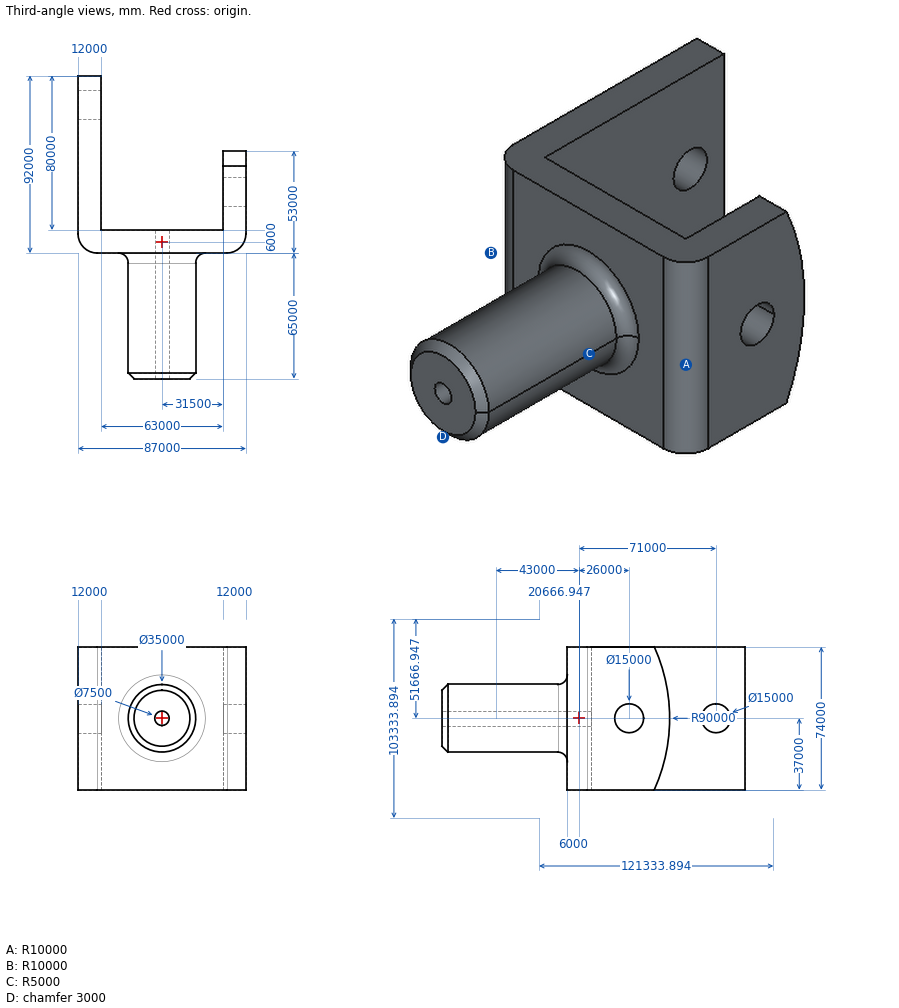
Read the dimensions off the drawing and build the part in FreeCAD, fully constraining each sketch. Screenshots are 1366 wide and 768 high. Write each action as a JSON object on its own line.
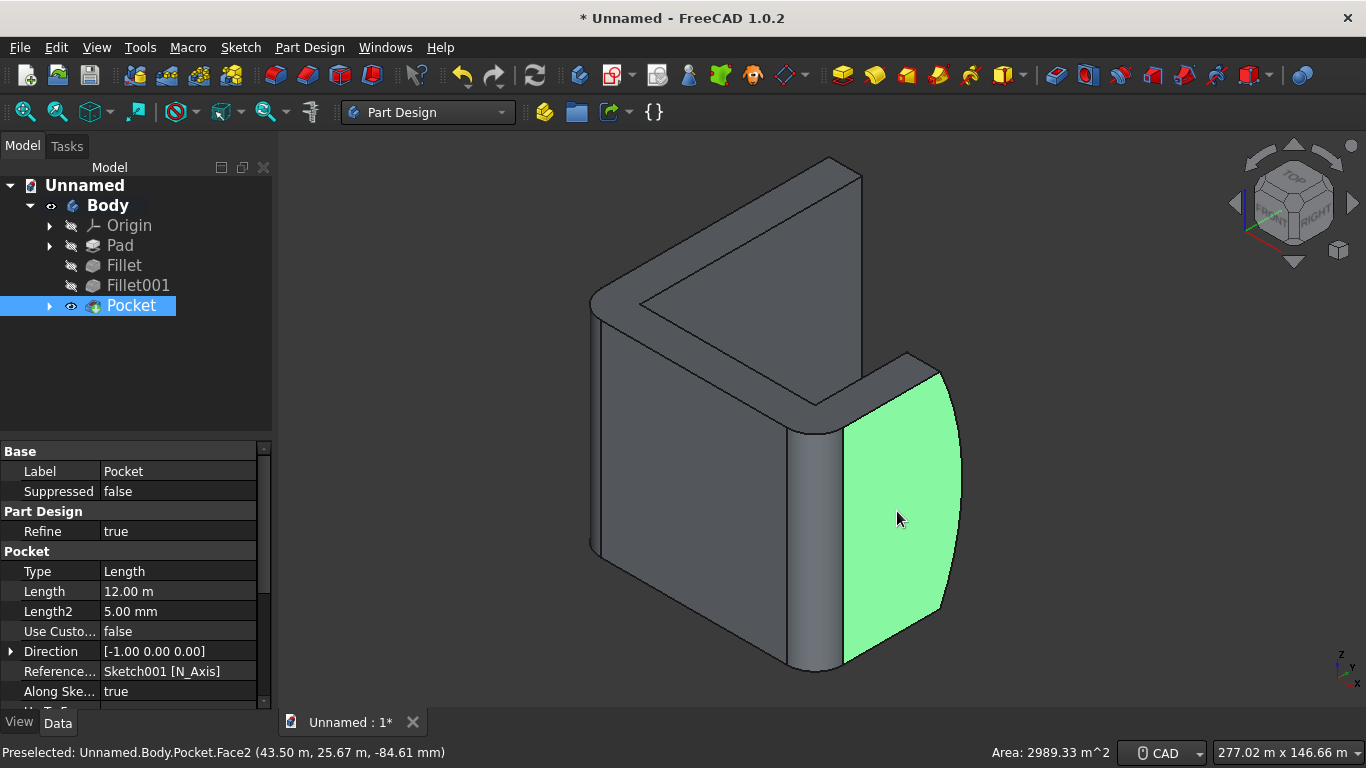
{"action": "left_click", "coordinate": [612, 76]}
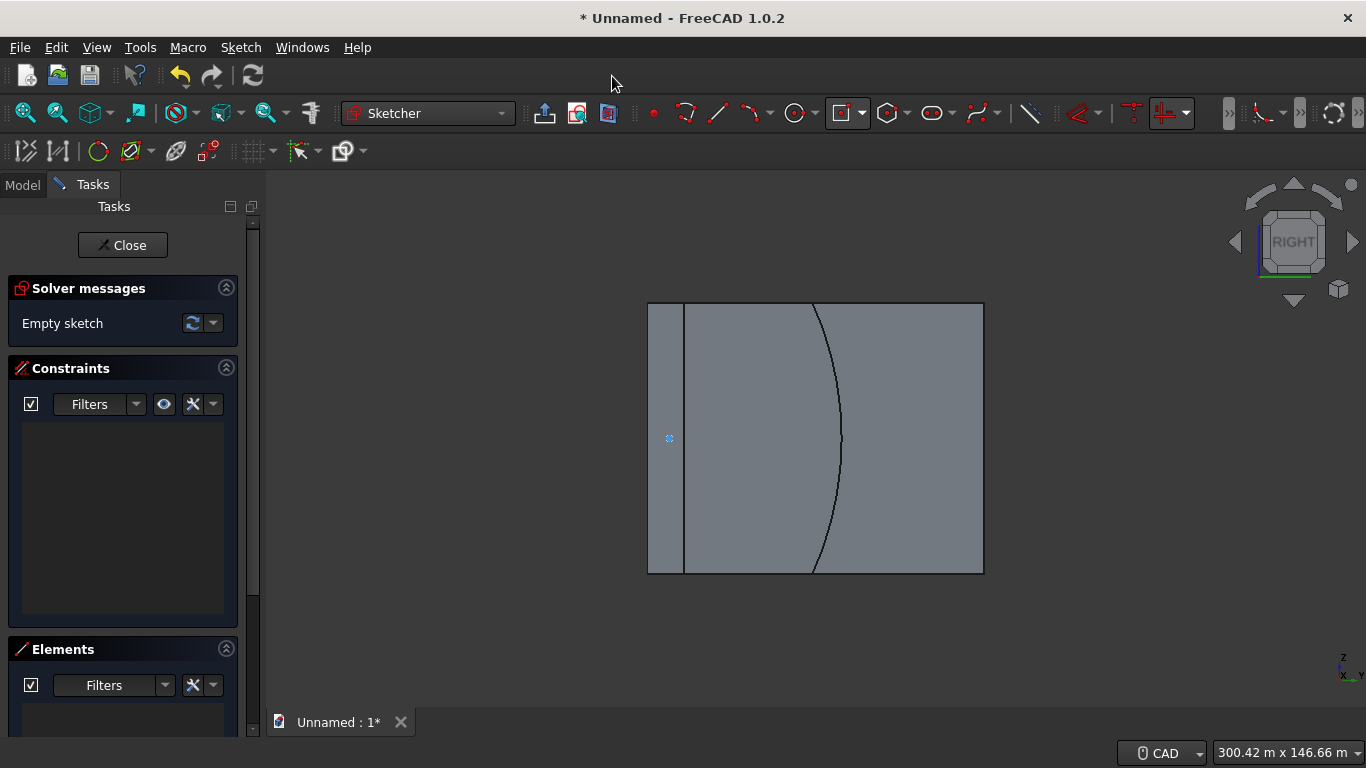
{"action": "scroll", "coordinate": [727, 438], "scroll_direction": "up", "scroll_amount": 8}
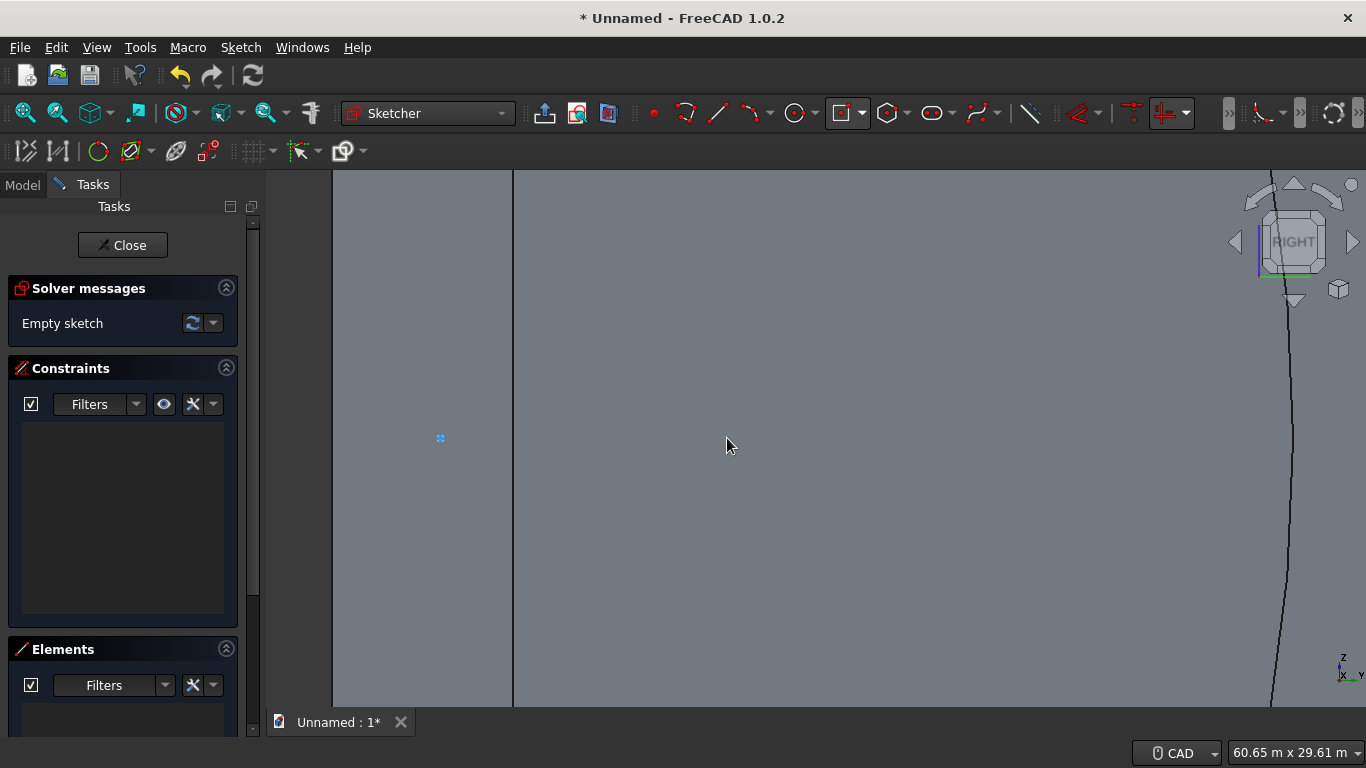
{"action": "left_click", "coordinate": [796, 114]}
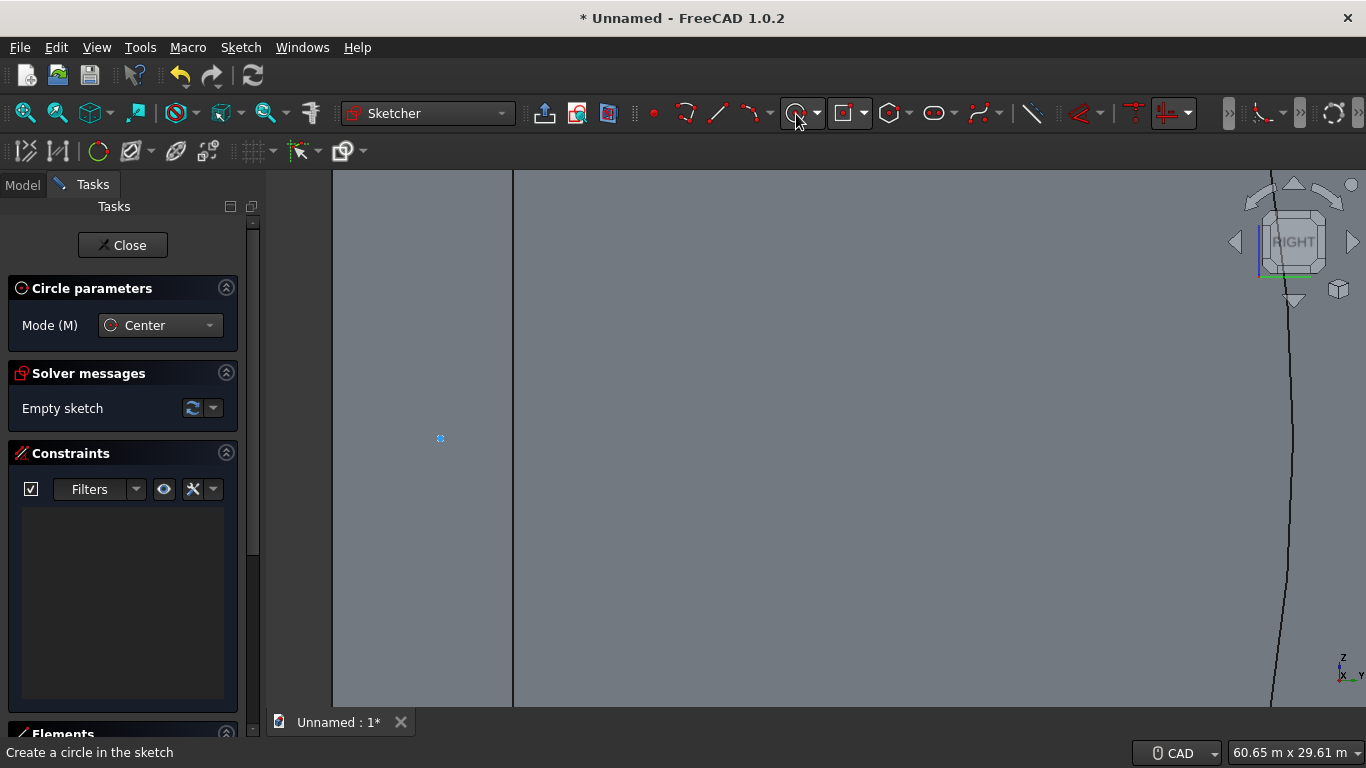
{"action": "left_click", "coordinate": [912, 438]}
{"action": "left_click", "coordinate": [1008, 342]}
{"action": "key", "text": "Escape"}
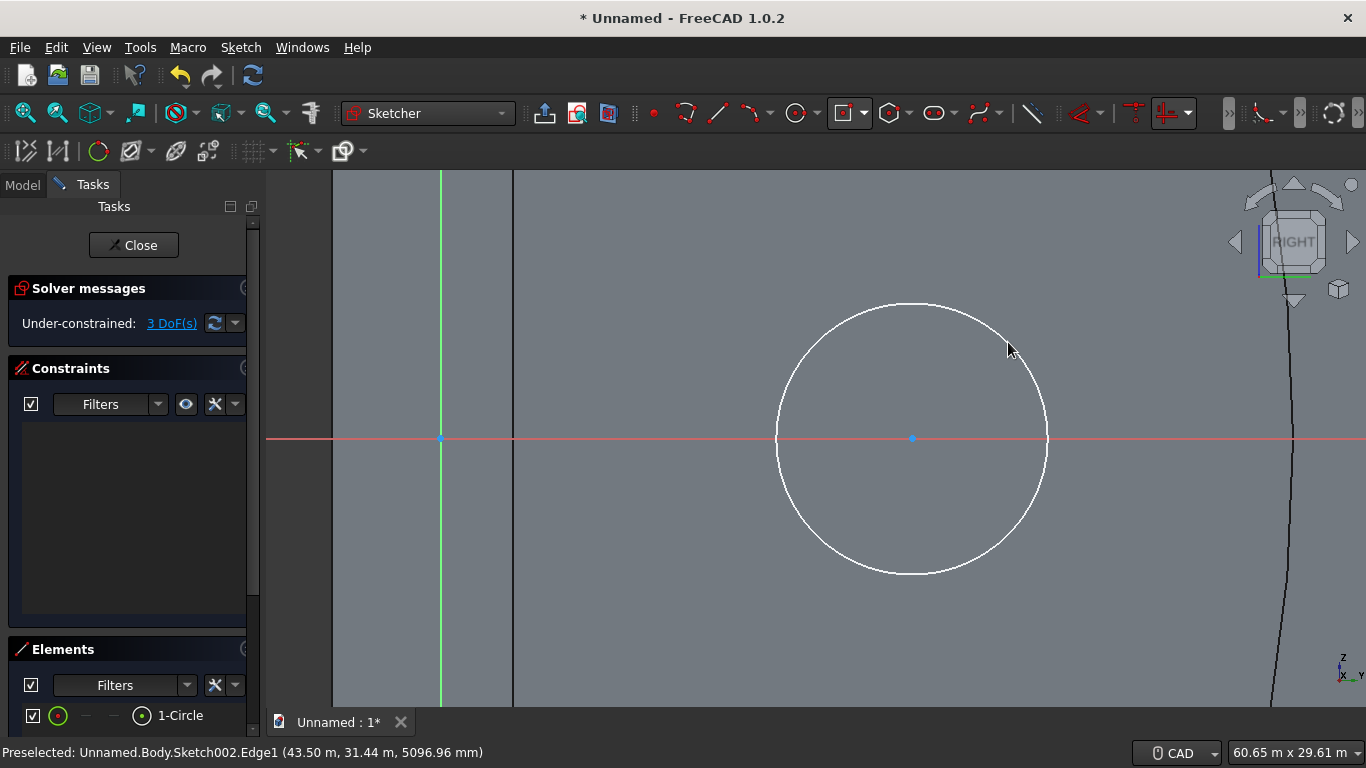
{"action": "left_click", "coordinate": [912, 439]}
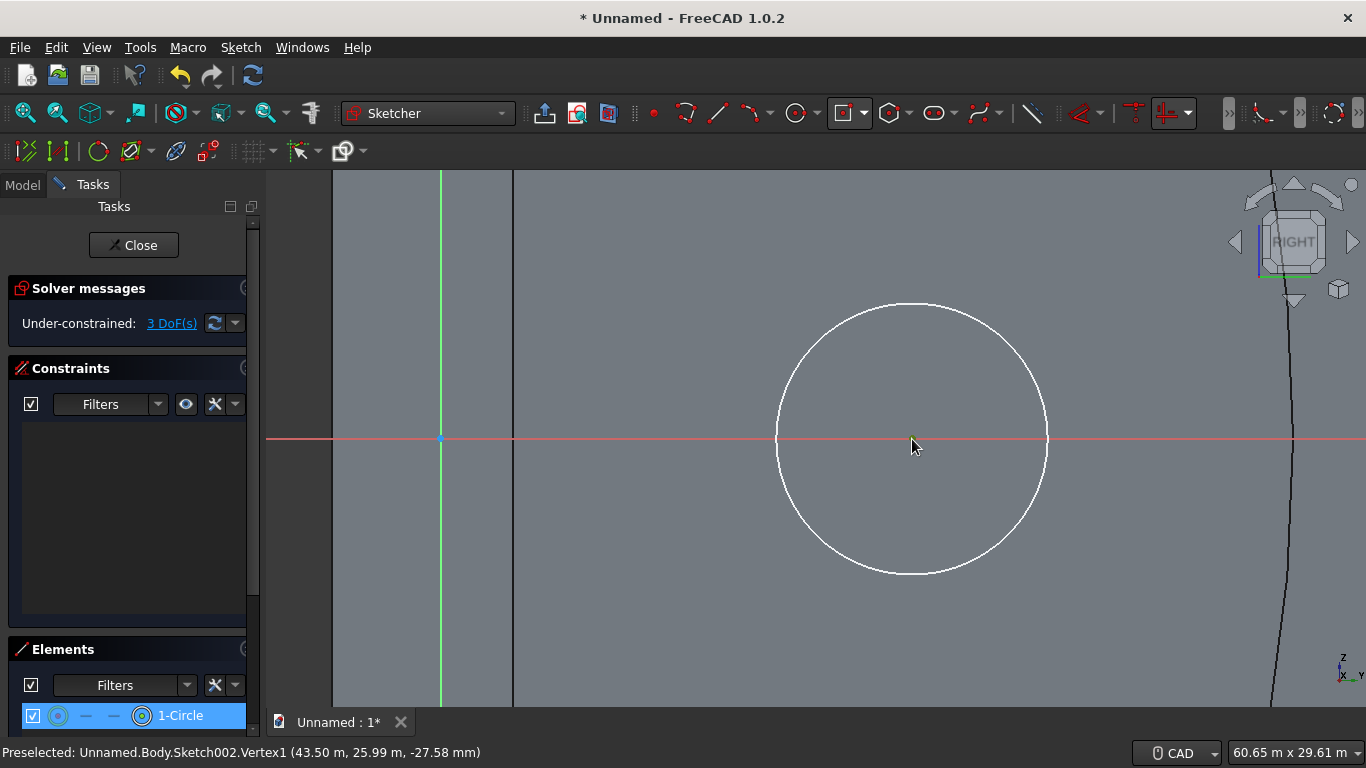
{"action": "left_click", "coordinate": [359, 438]}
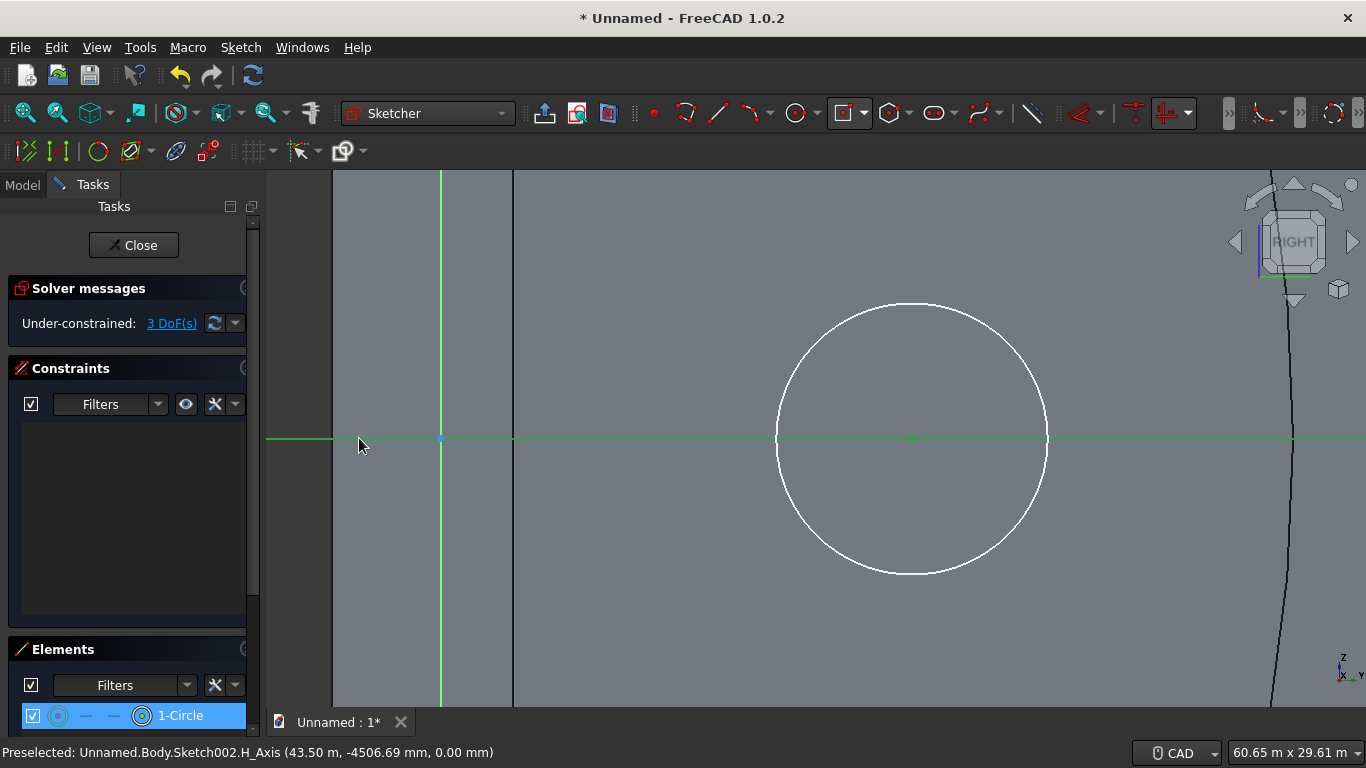
{"action": "left_click", "coordinate": [1134, 114]}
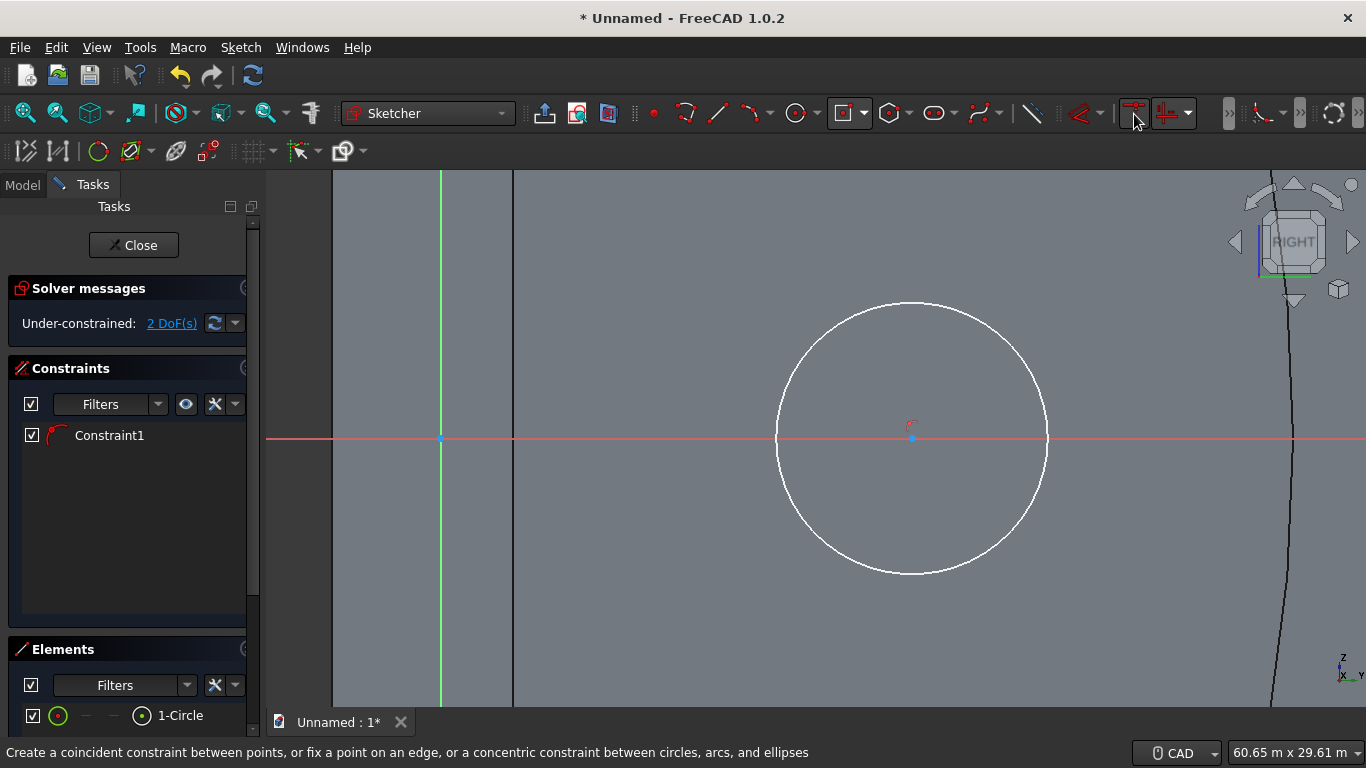
{"action": "left_click", "coordinate": [1080, 114]}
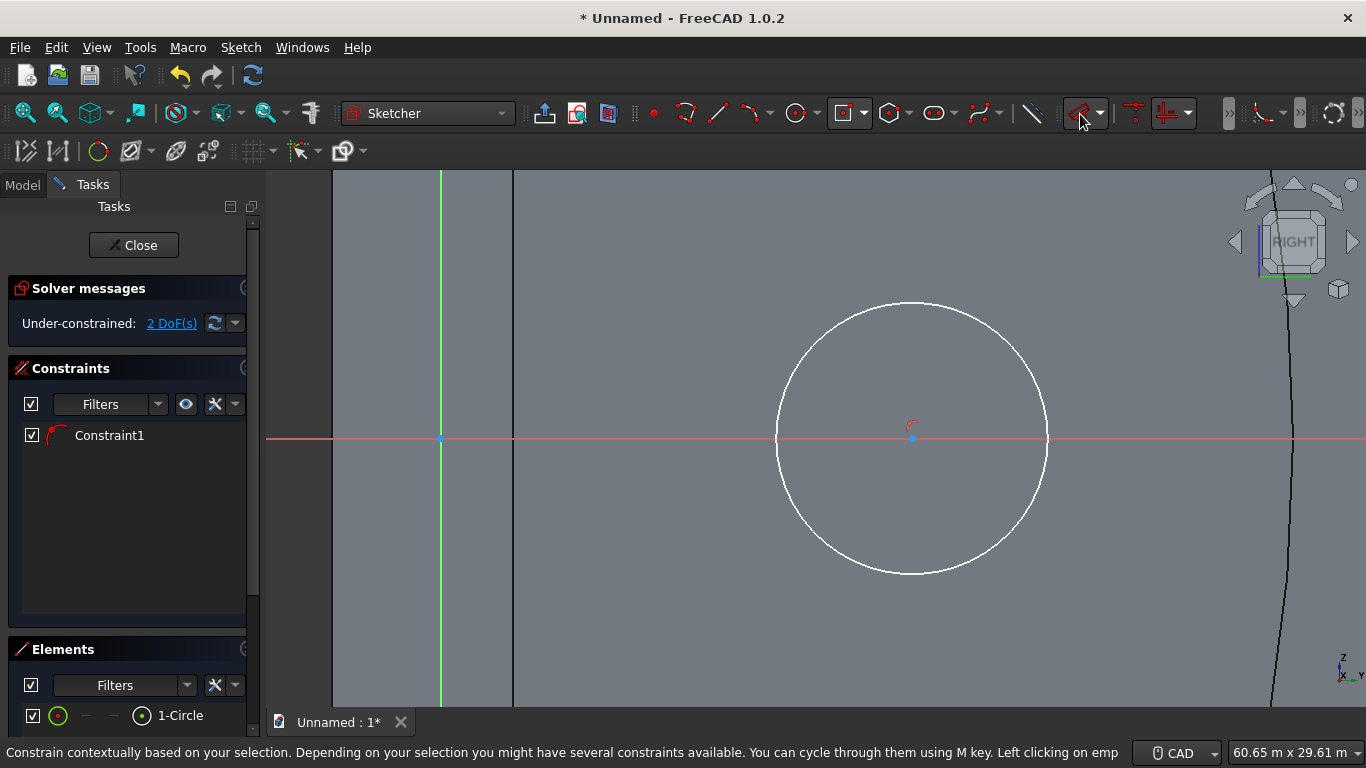
{"action": "left_click", "coordinate": [1008, 342]}
{"action": "left_click", "coordinate": [1031, 319]}